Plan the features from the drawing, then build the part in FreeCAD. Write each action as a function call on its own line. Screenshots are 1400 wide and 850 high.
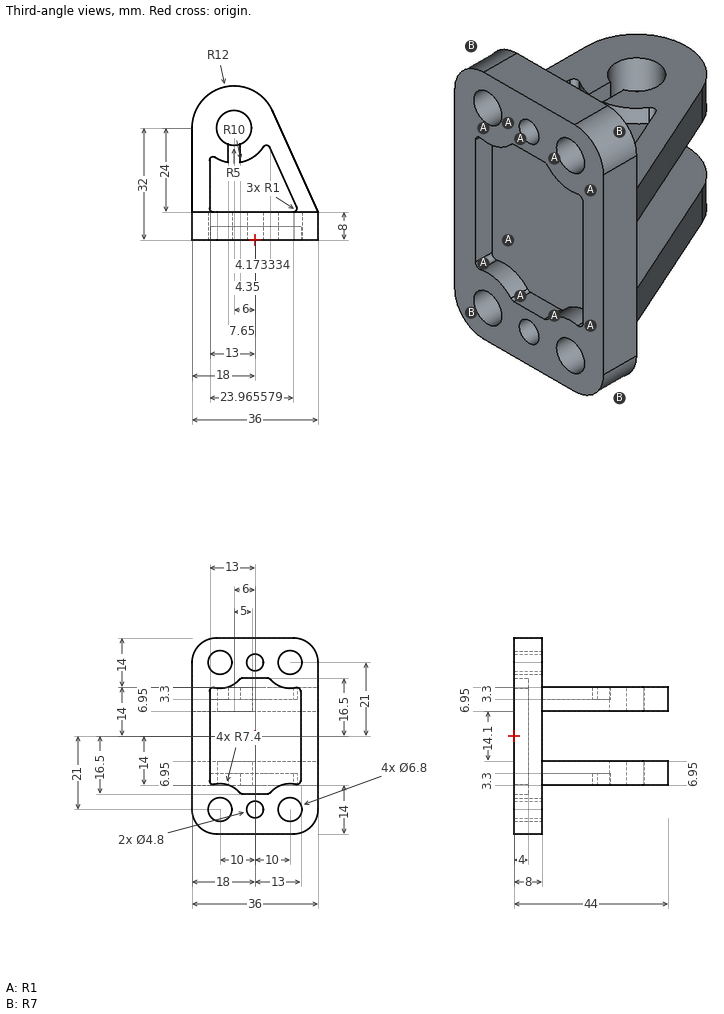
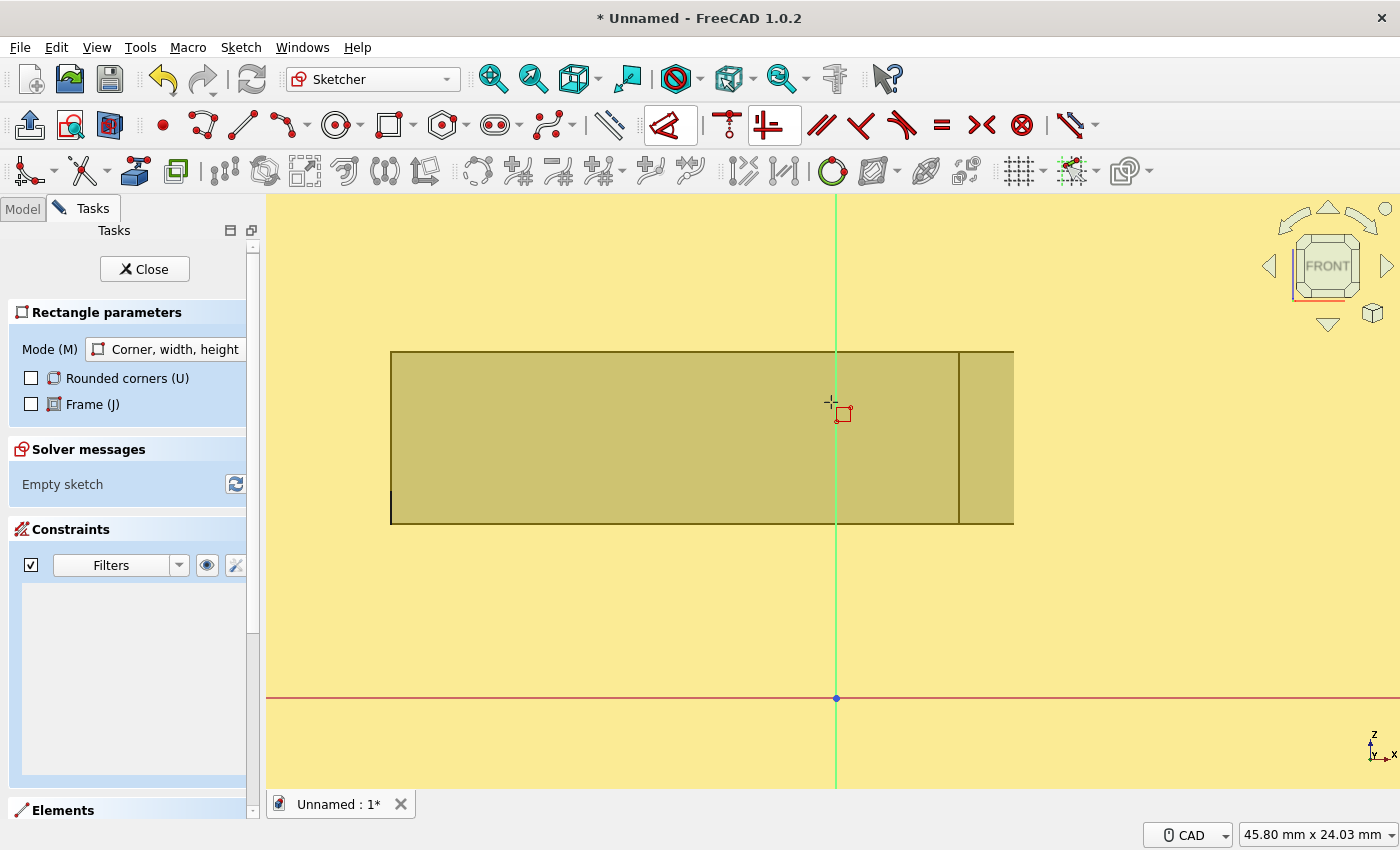
click(688, 352)
move(812, 524)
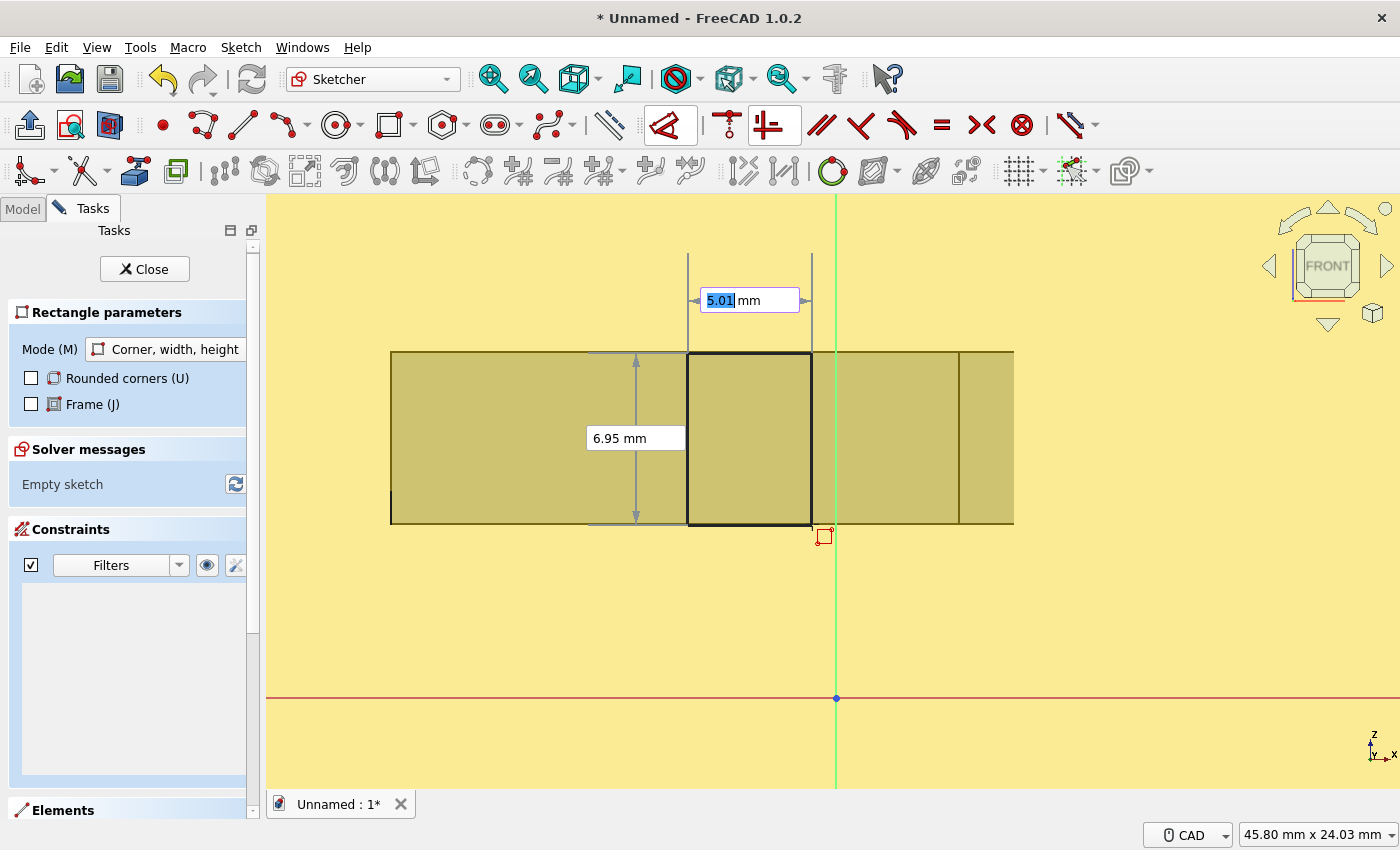
text(5)
key(Tab)
text(6.95)
key(Return)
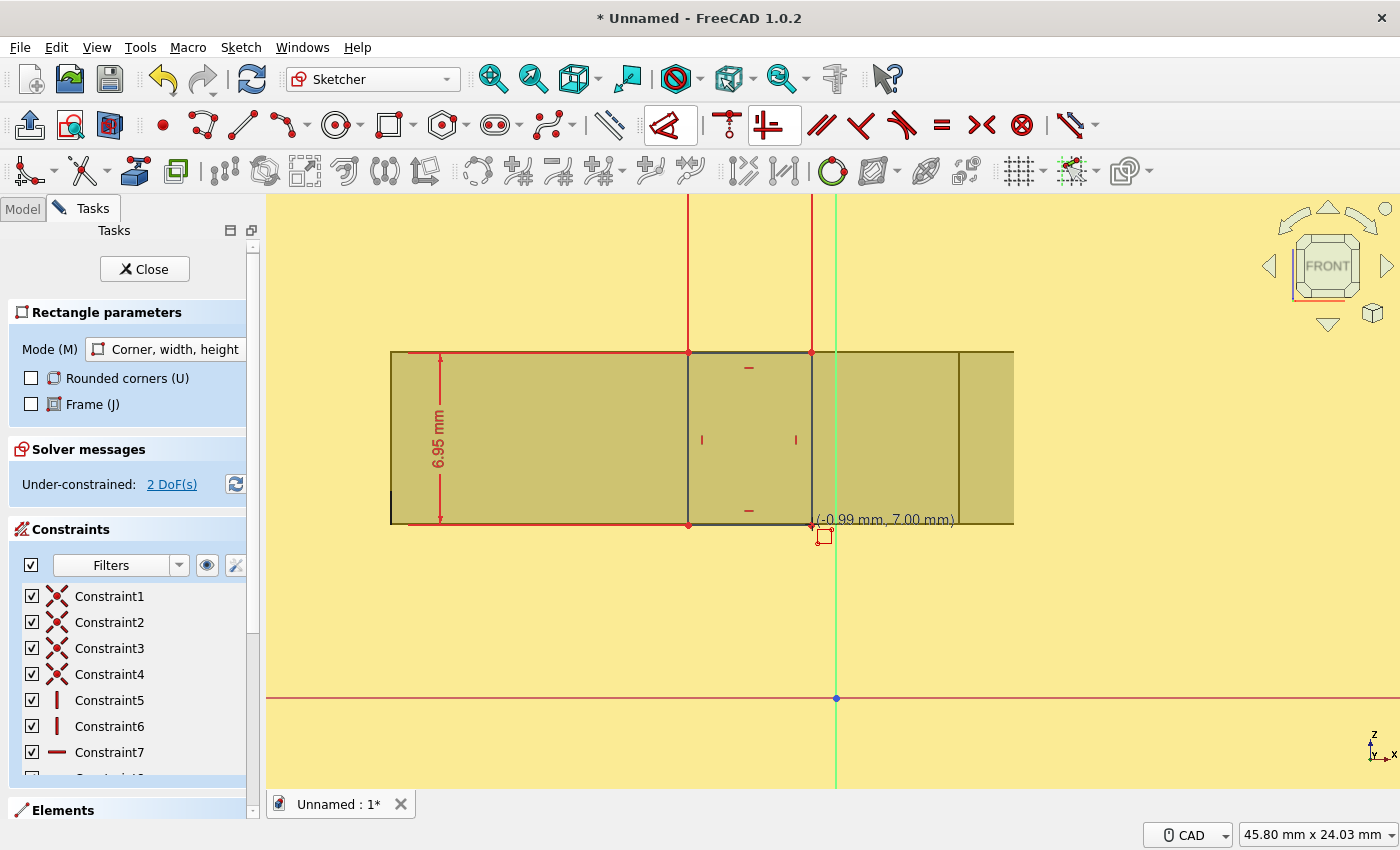
click(244, 126)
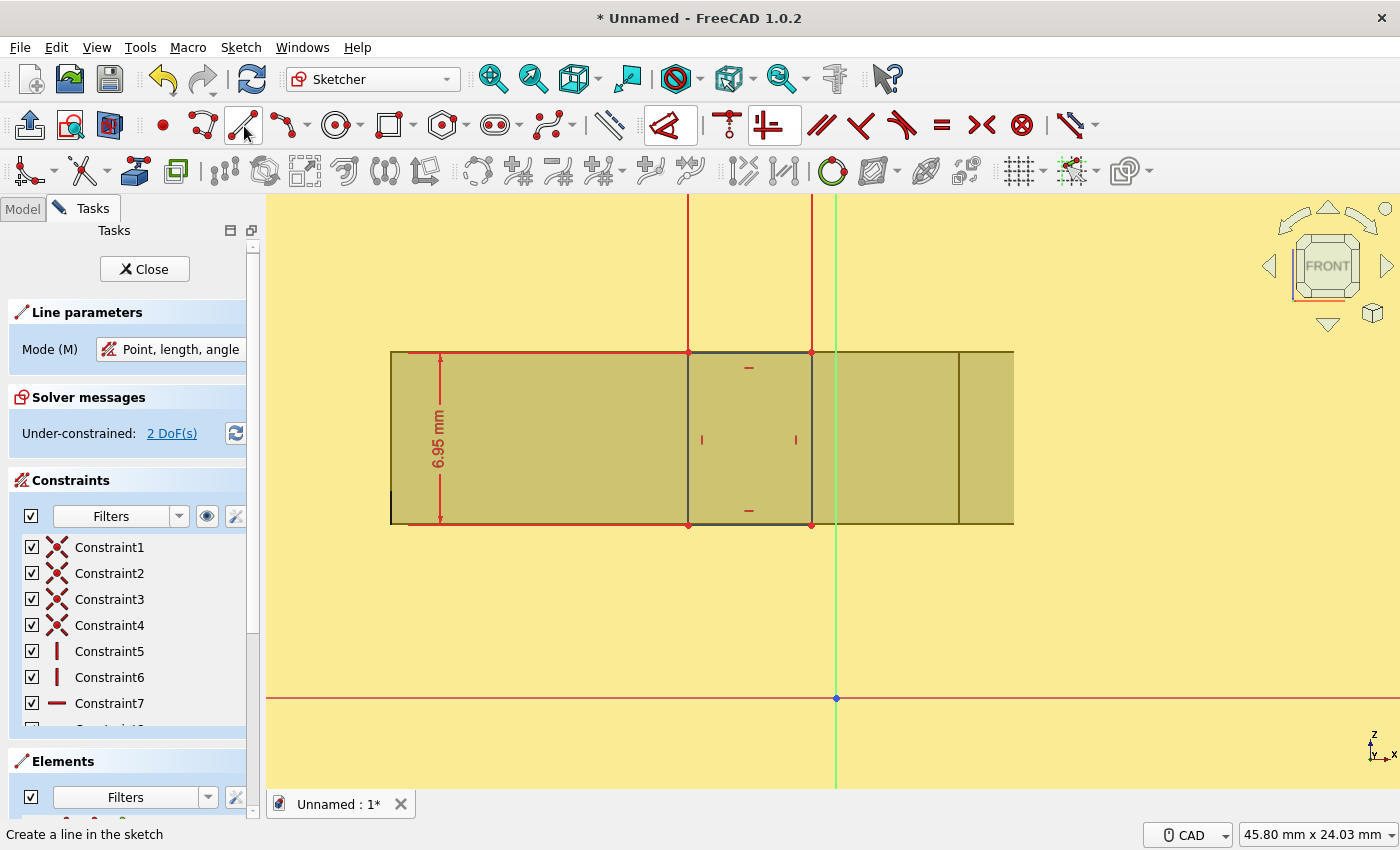
click(688, 335)
click(688, 283)
key(Escape)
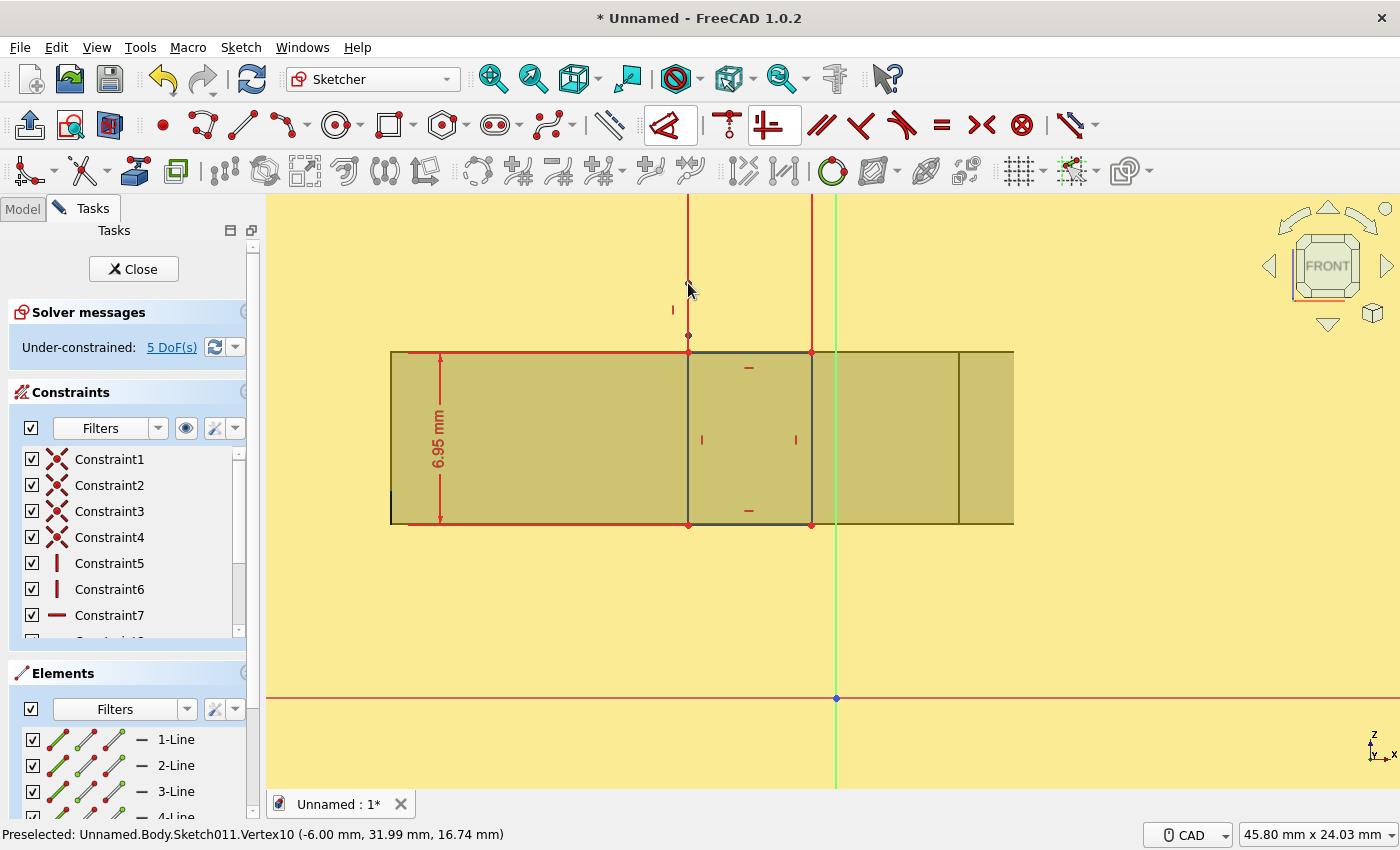
click(688, 320)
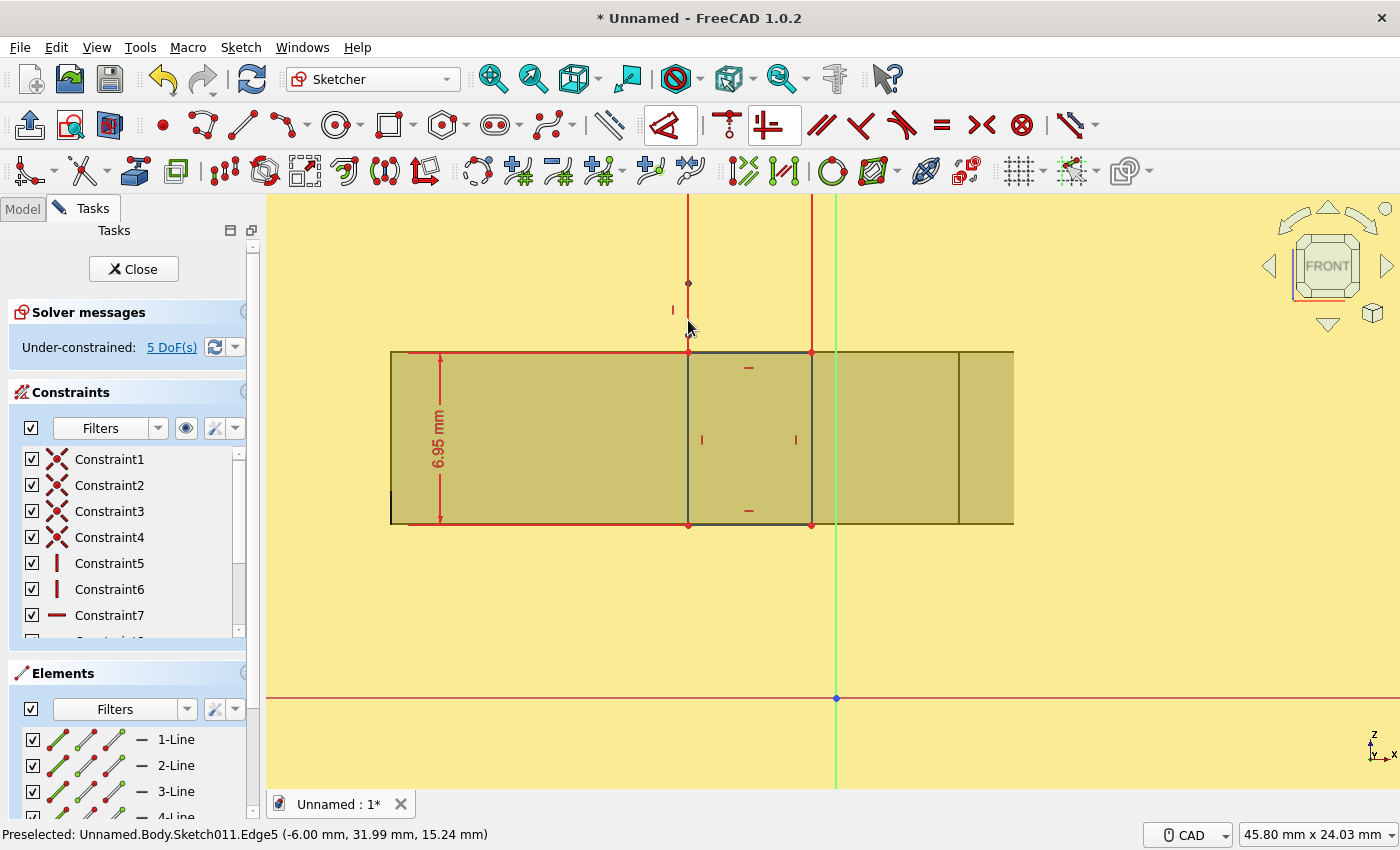
key(g)
key(n)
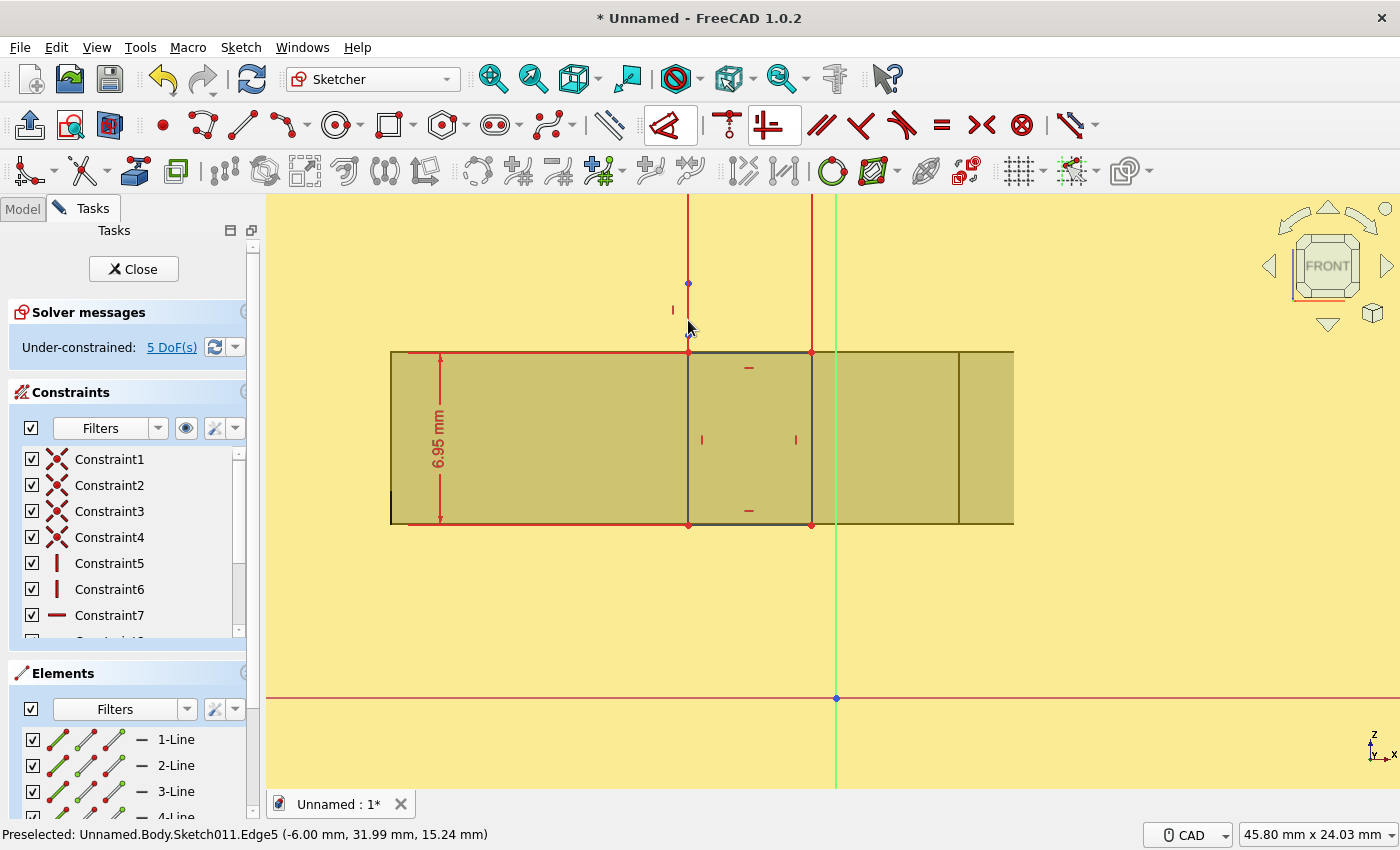
click(688, 353)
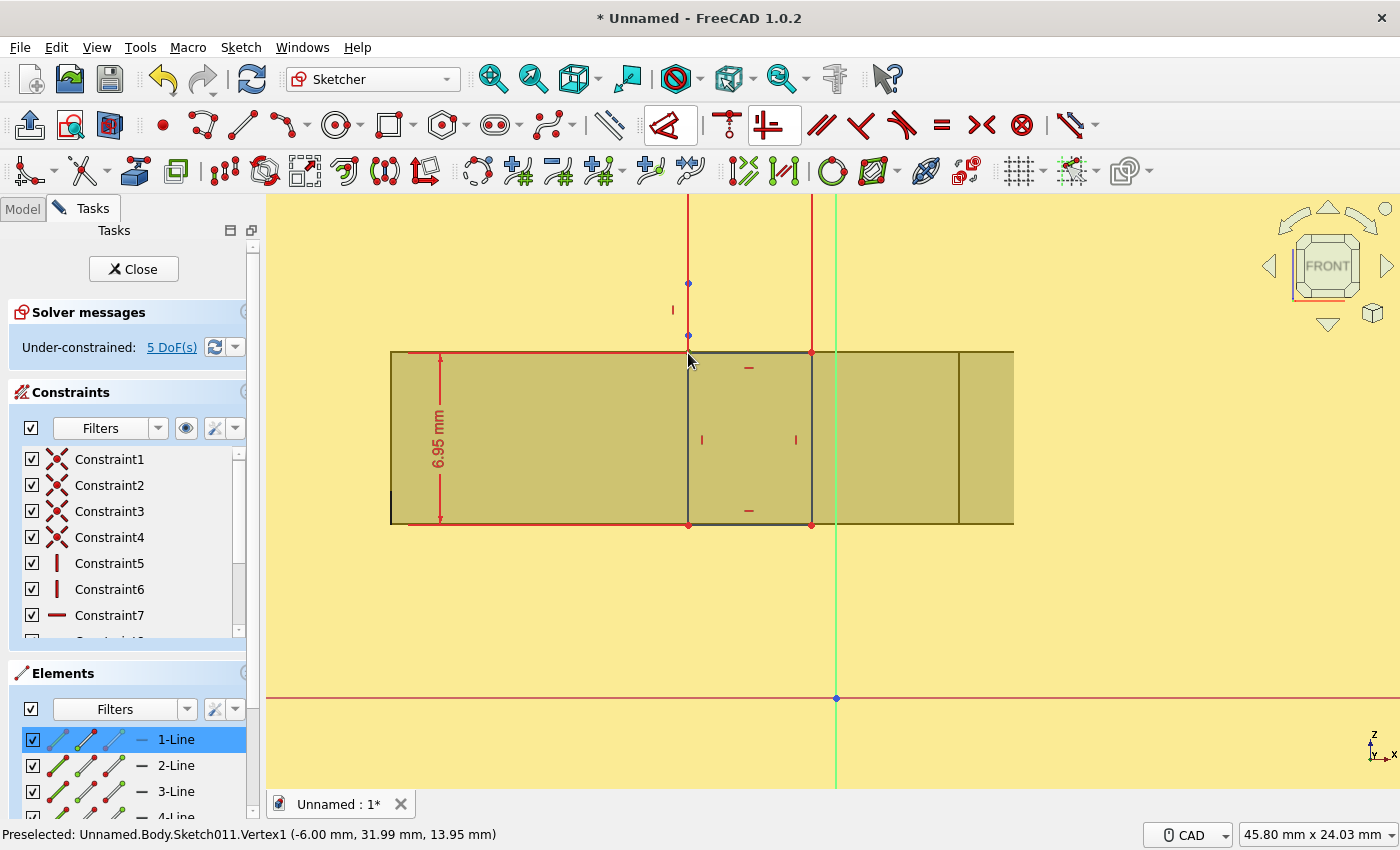
key(l)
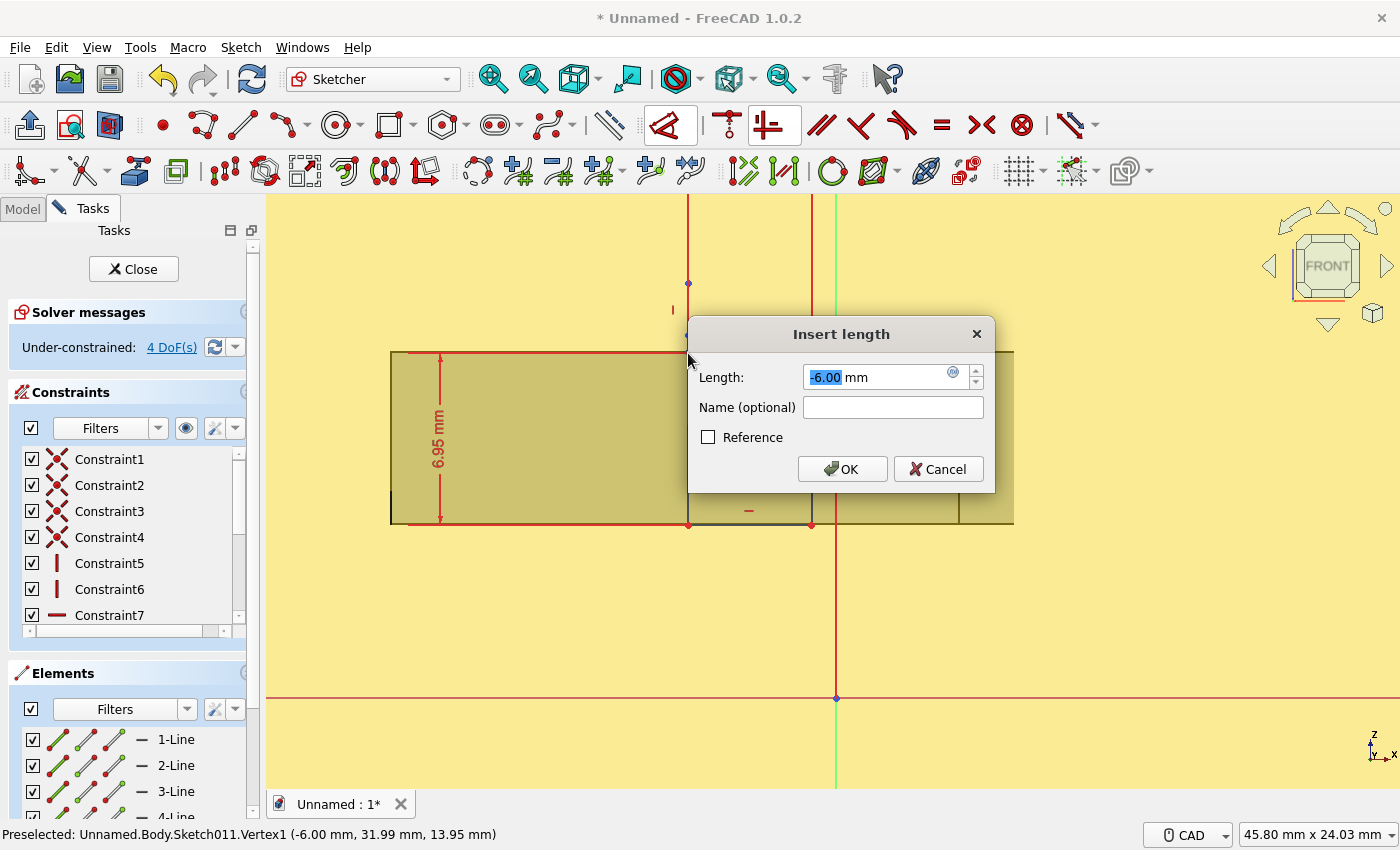
text(-6)
key(Return)